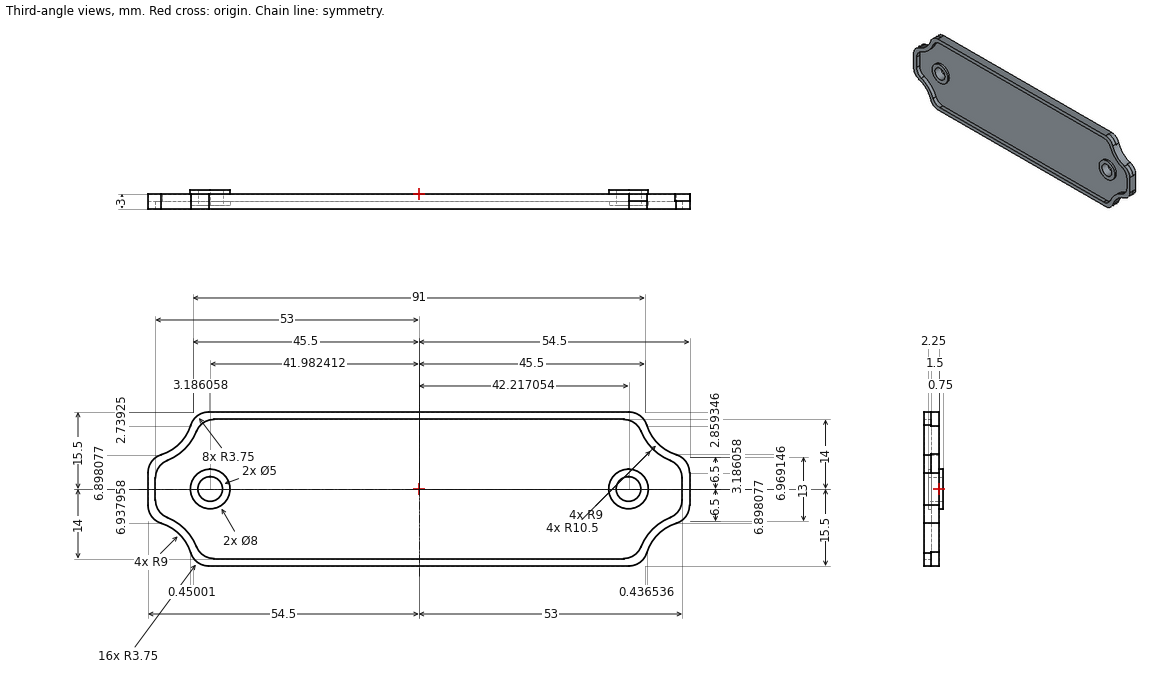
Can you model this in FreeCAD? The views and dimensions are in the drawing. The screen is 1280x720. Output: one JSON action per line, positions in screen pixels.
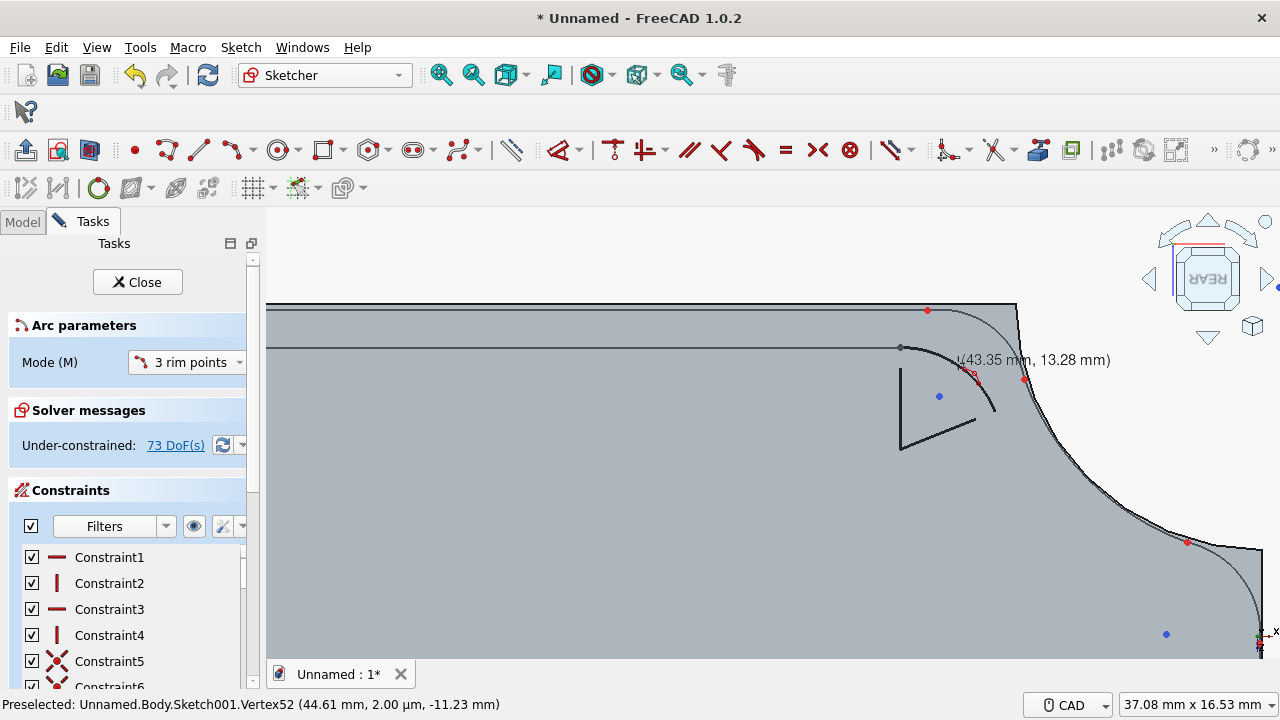
{"action": "left_click", "coordinate": [957, 363]}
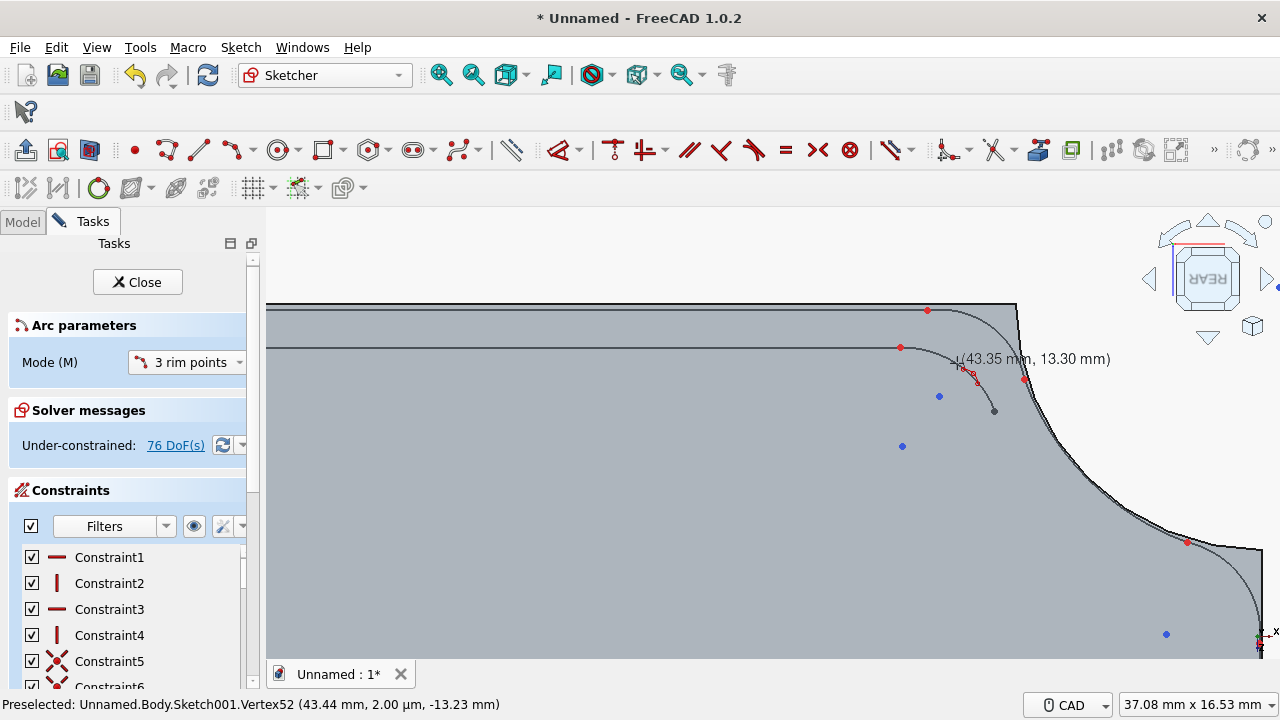
{"action": "left_click", "coordinate": [995, 412]}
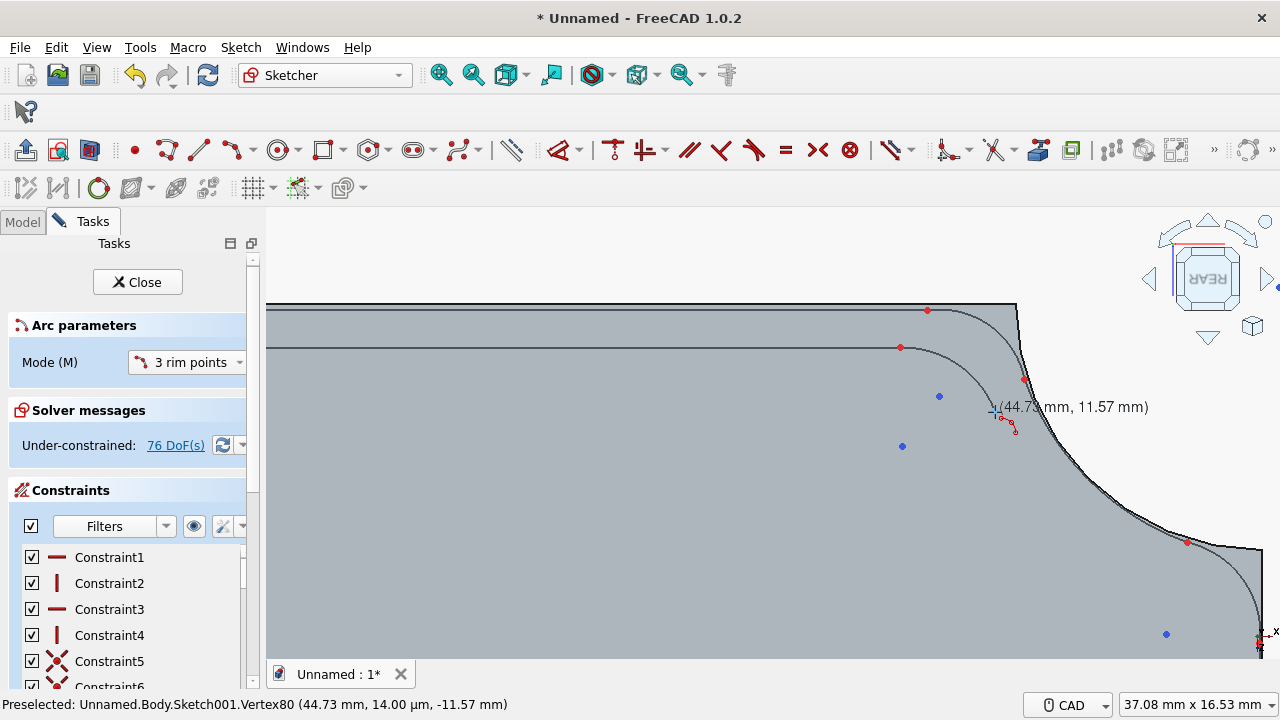
{"action": "scroll", "coordinate": [940, 358], "scroll_direction": "down", "scroll_amount": 8}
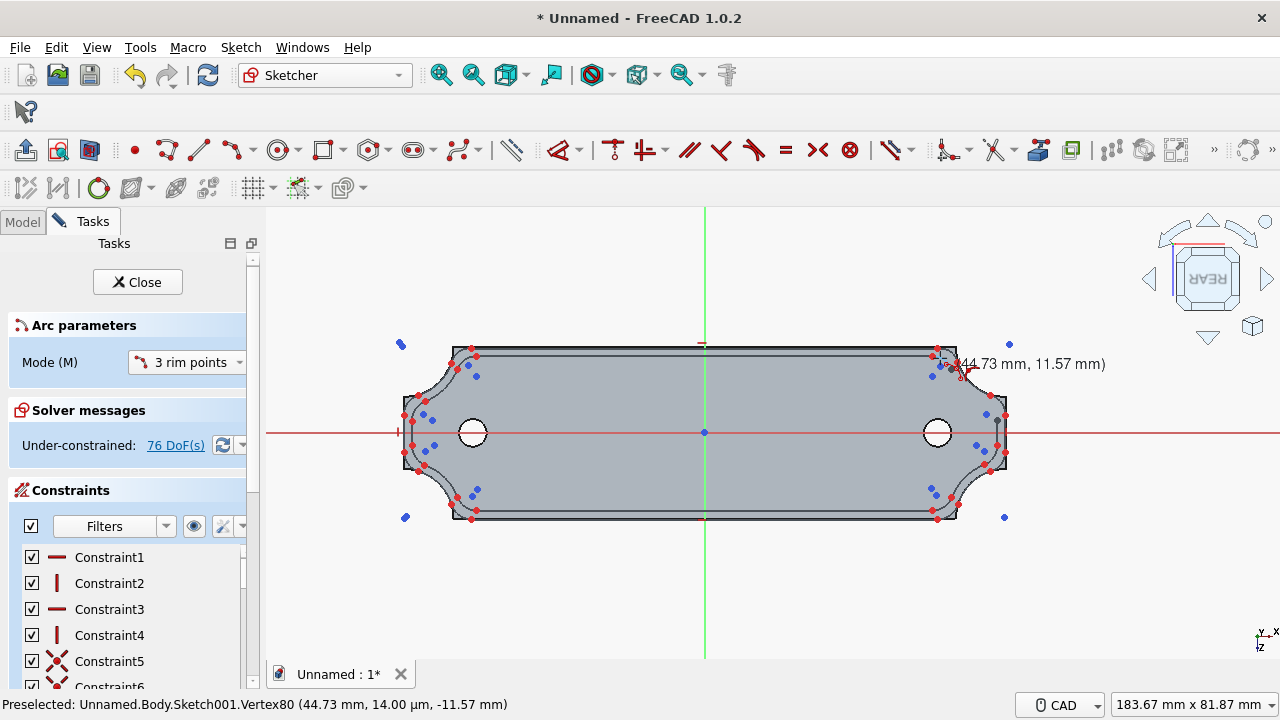
{"action": "scroll", "coordinate": [984, 401], "scroll_direction": "up", "scroll_amount": 4}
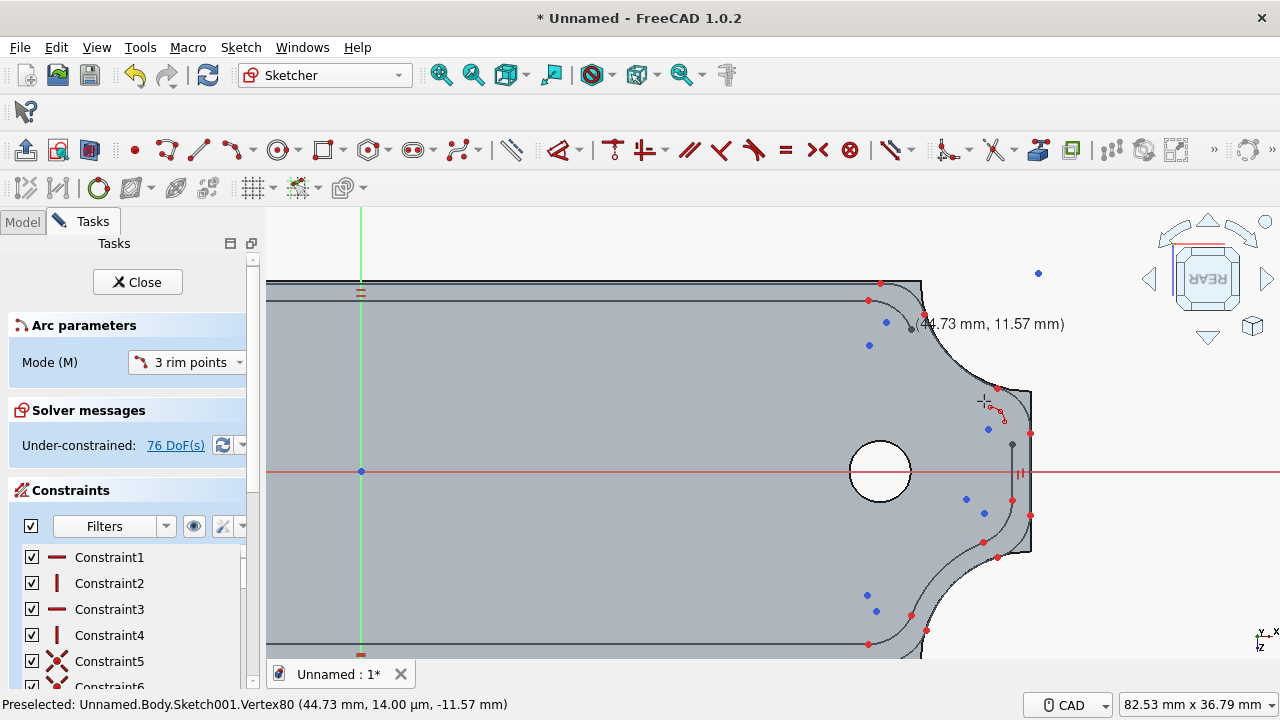
{"action": "left_click", "coordinate": [984, 401]}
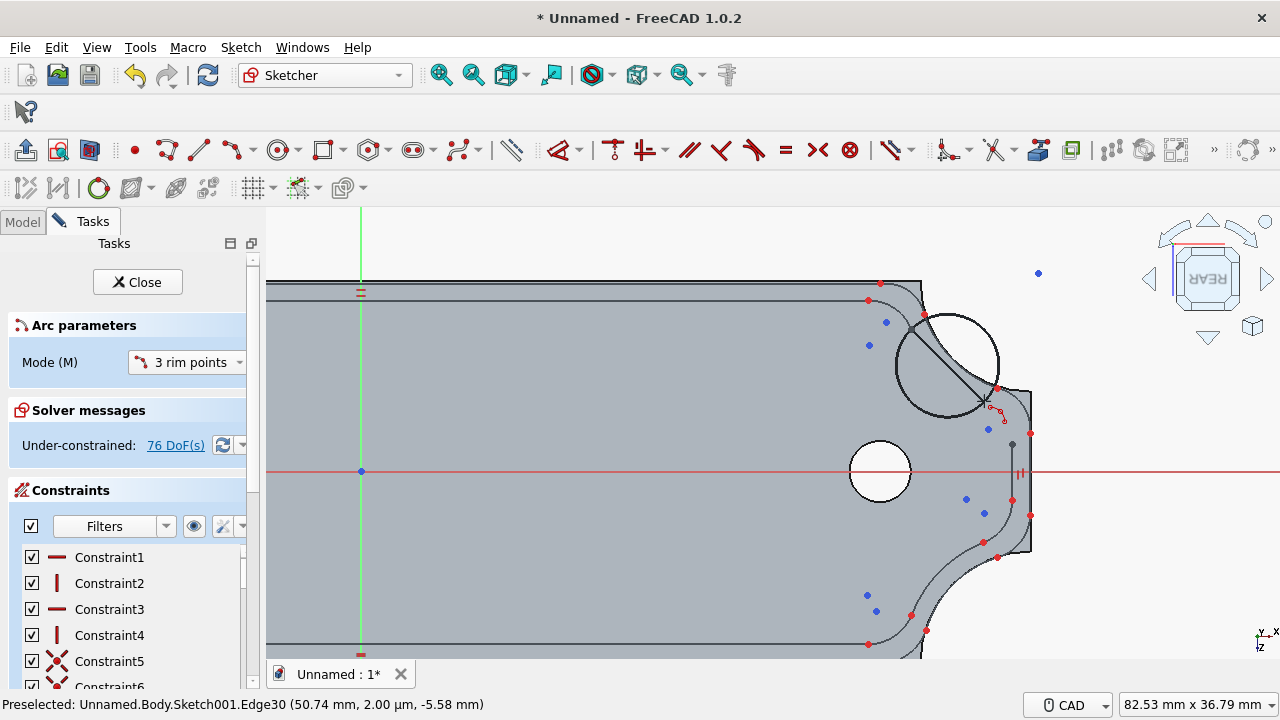
{"action": "scroll", "coordinate": [940, 372], "scroll_direction": "up", "scroll_amount": 3}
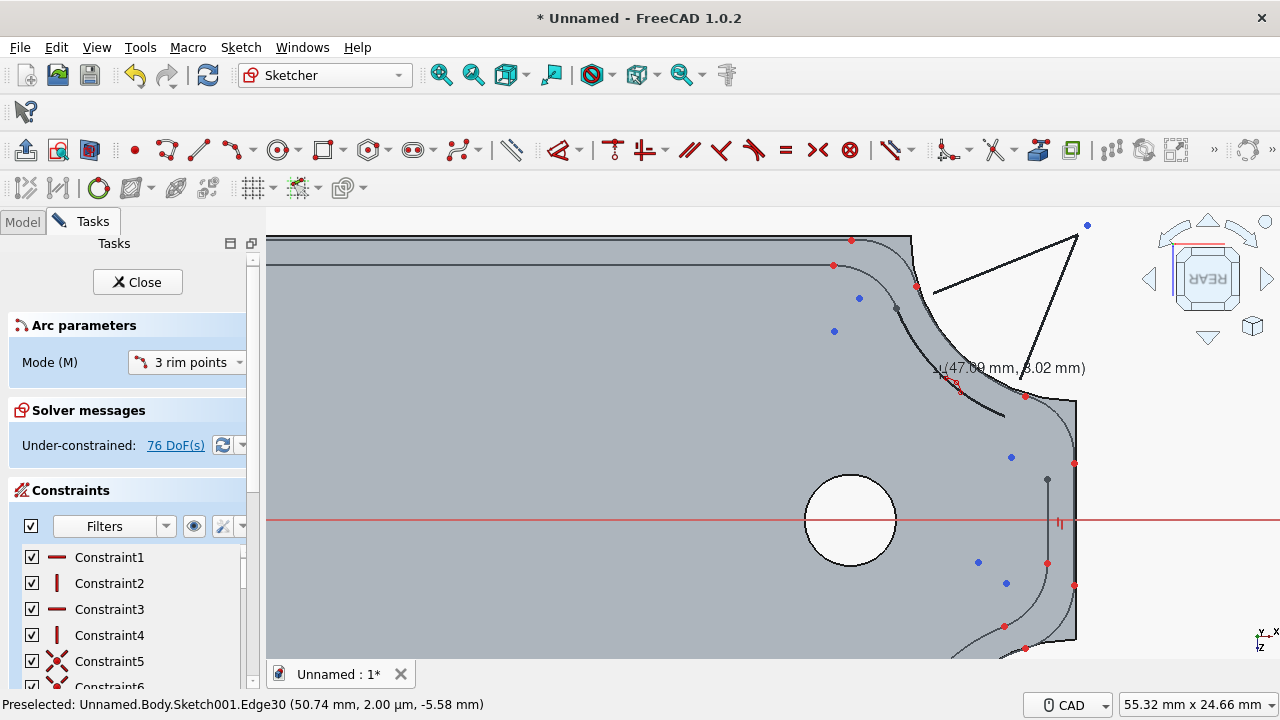
{"action": "left_click", "coordinate": [939, 372]}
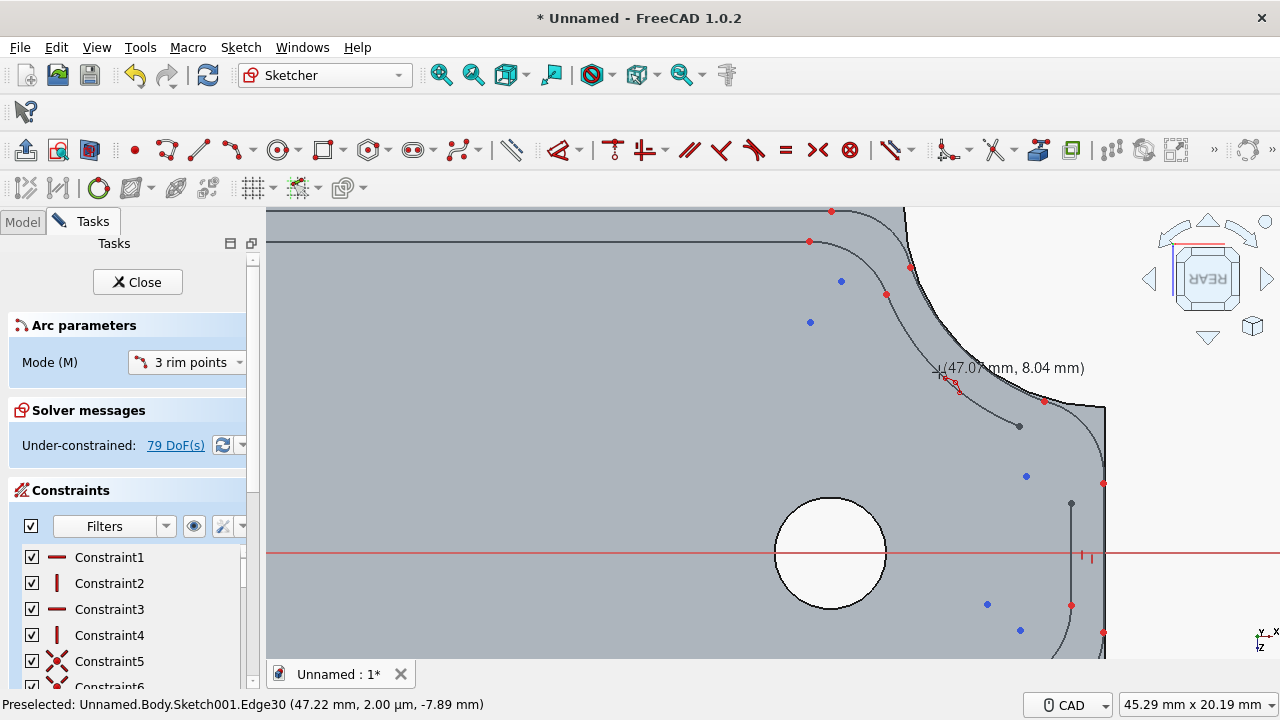
{"action": "left_click", "coordinate": [1020, 426]}
{"action": "left_click", "coordinate": [1071, 504]}
{"action": "left_click", "coordinate": [1057, 455]}
{"action": "key", "text": "Escape"}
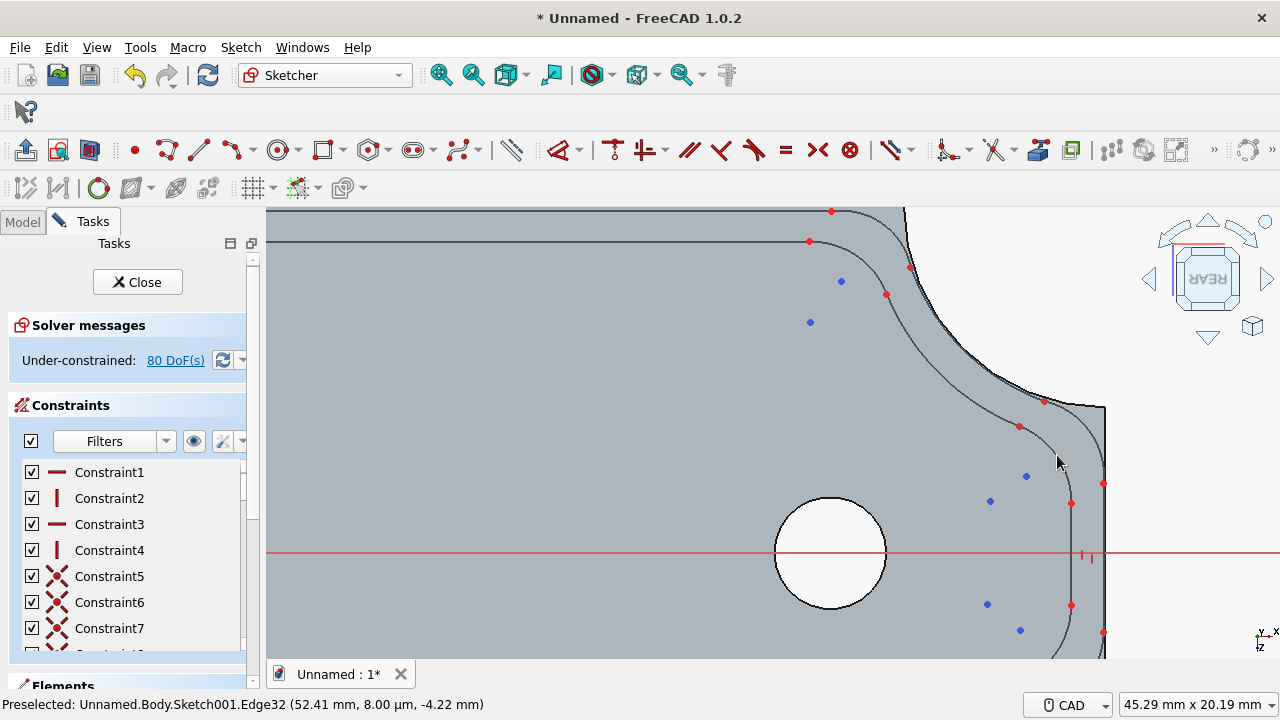
{"action": "scroll", "coordinate": [973, 394], "scroll_direction": "down", "scroll_amount": 7}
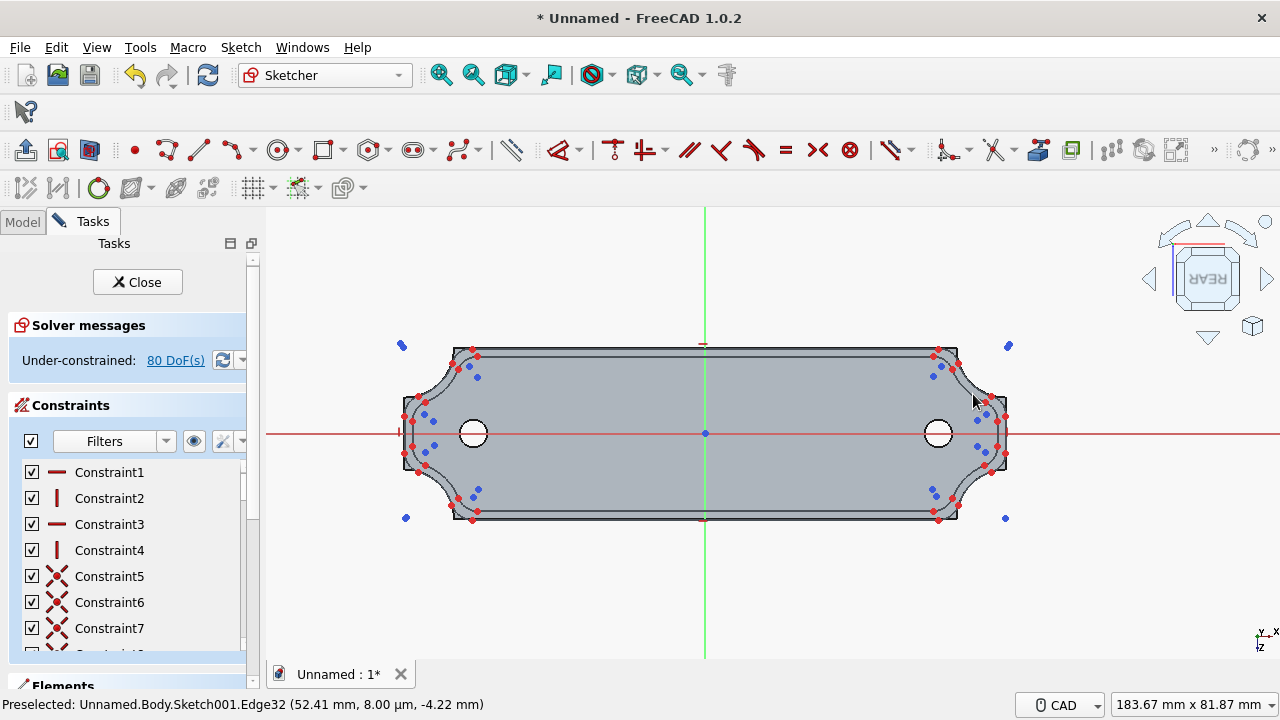
{"action": "scroll", "coordinate": [799, 349], "scroll_direction": "up", "scroll_amount": 4}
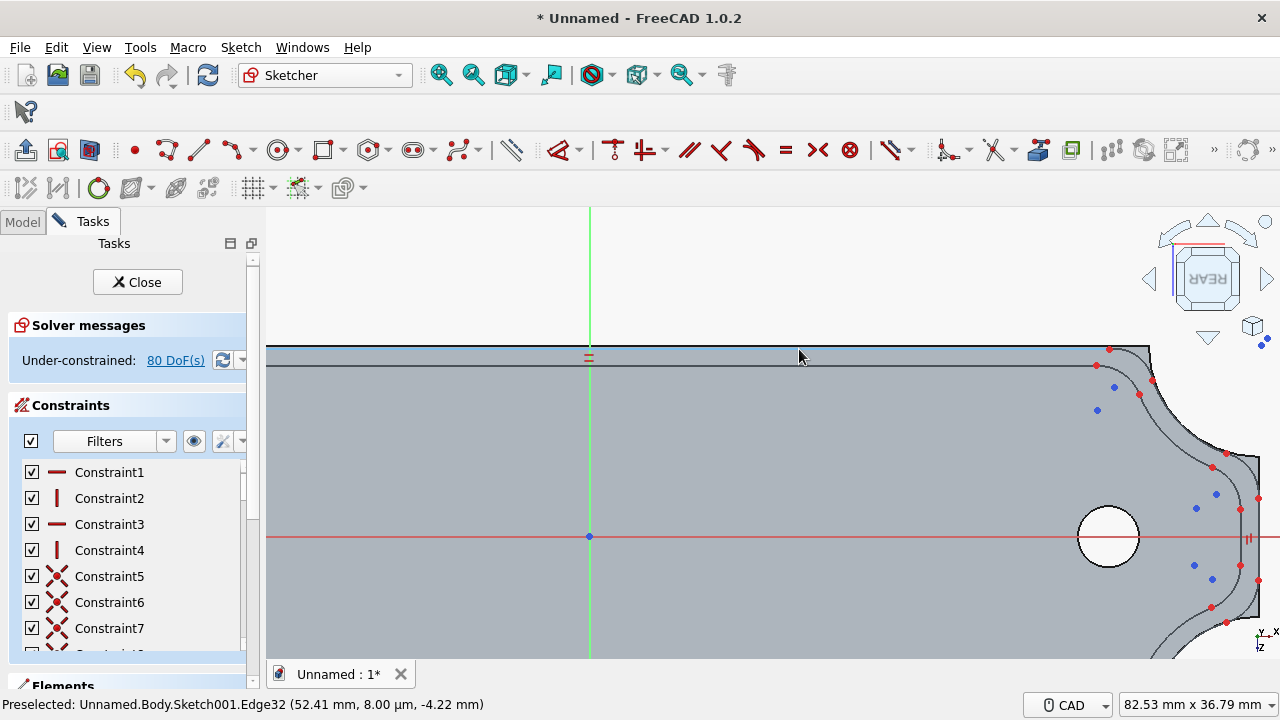
{"action": "left_click", "coordinate": [797, 349]}